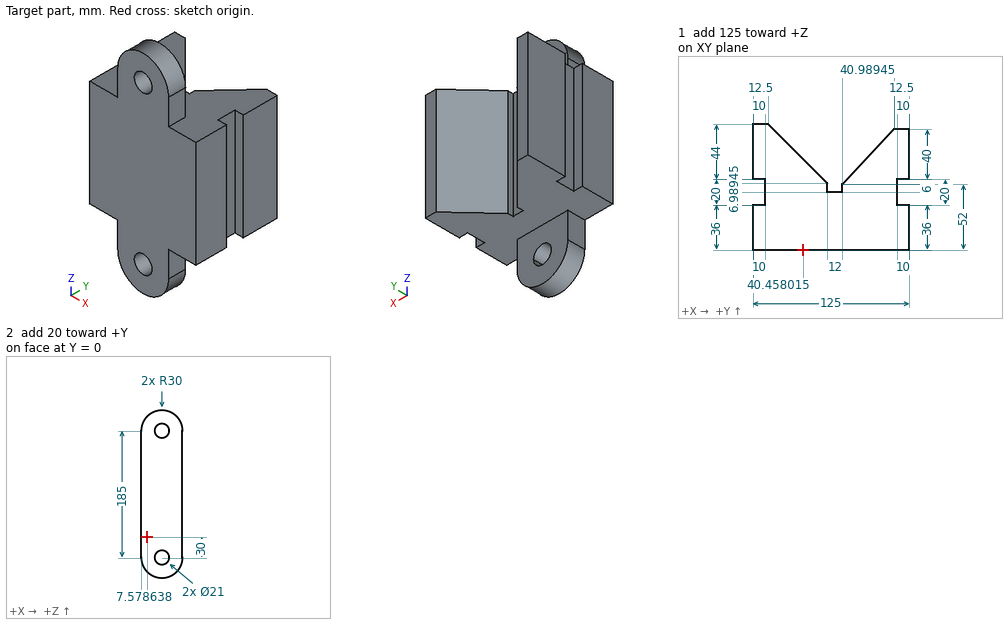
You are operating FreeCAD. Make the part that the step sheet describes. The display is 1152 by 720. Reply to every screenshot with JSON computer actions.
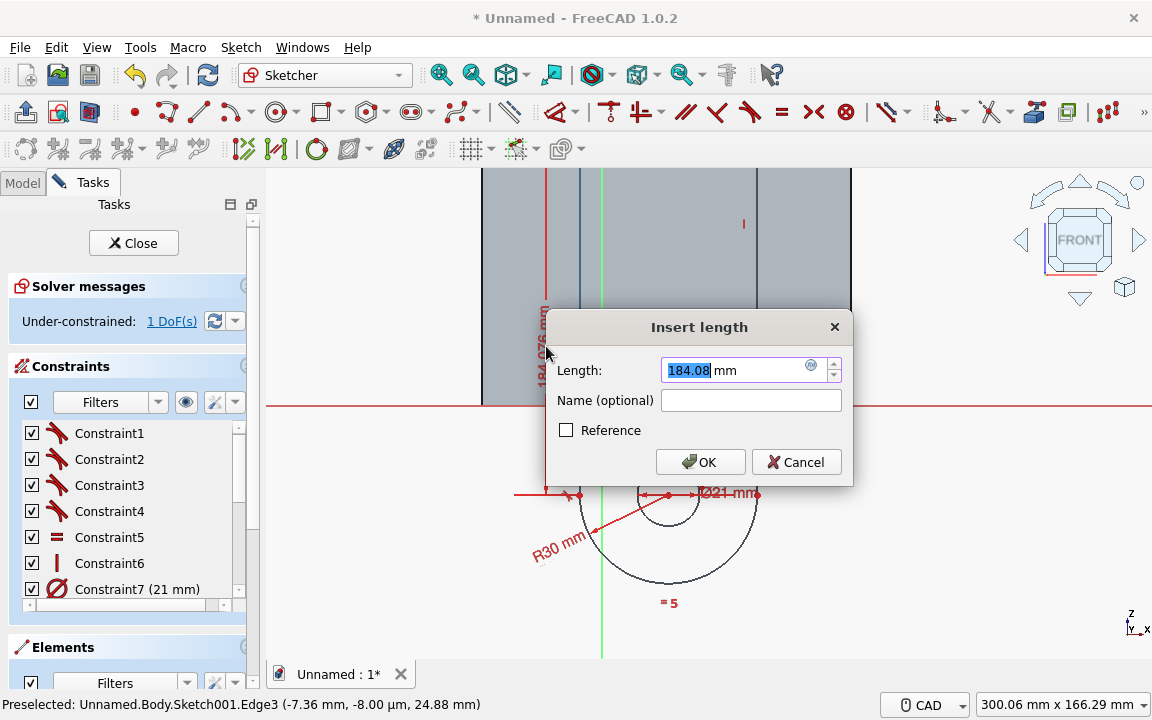
{"action": "type", "text": "185"}
{"action": "key", "text": "Return"}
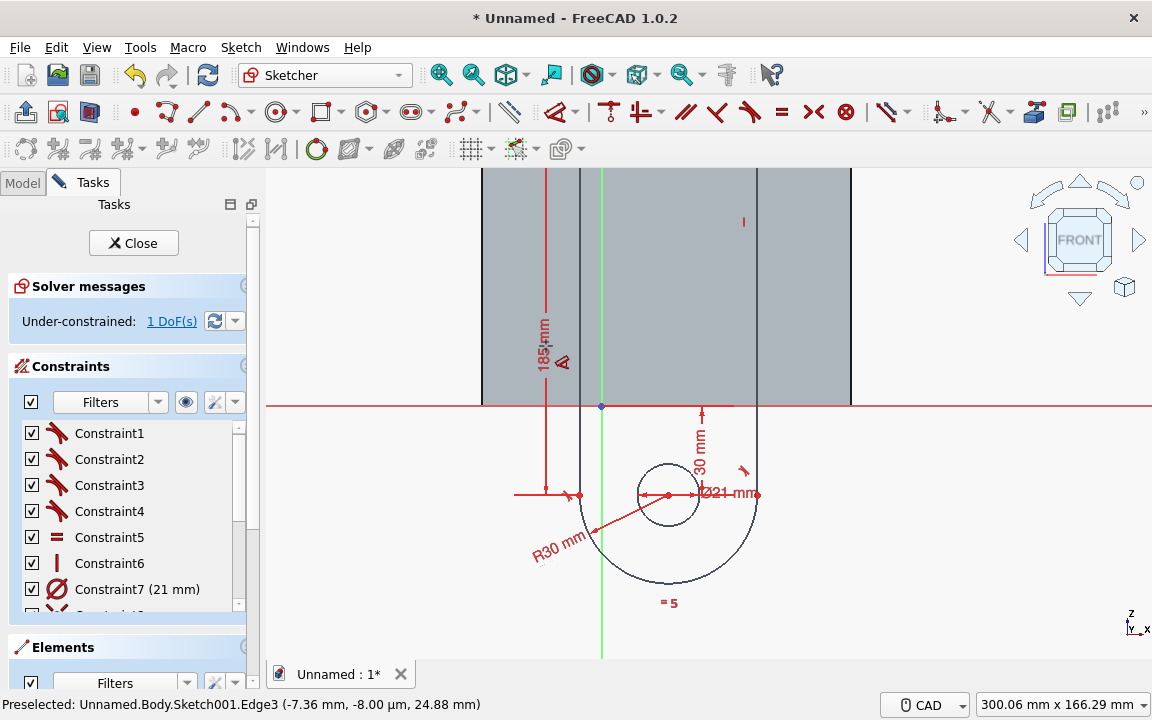
{"action": "scroll", "coordinate": [580, 495], "scroll_direction": "up", "scroll_amount": 3}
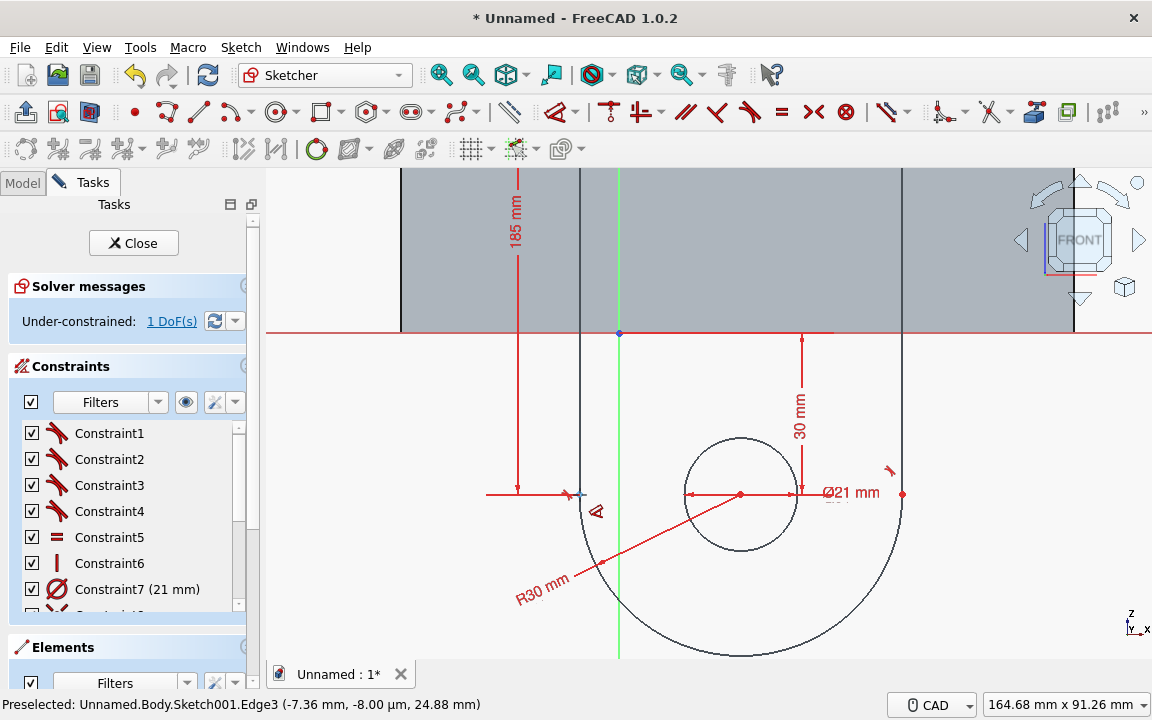
{"action": "left_click", "coordinate": [580, 495]}
{"action": "left_click", "coordinate": [599, 529]}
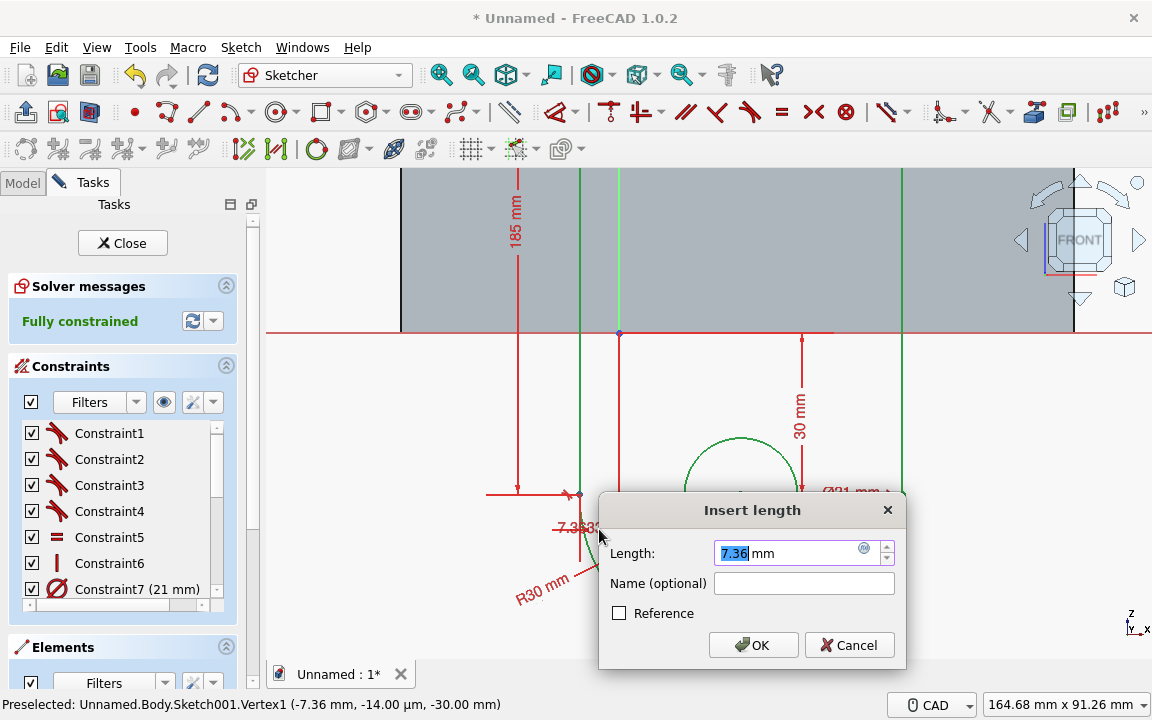
{"action": "type", "text": "7.578638"}
{"action": "key", "text": "Return"}
{"action": "key", "text": "Escape"}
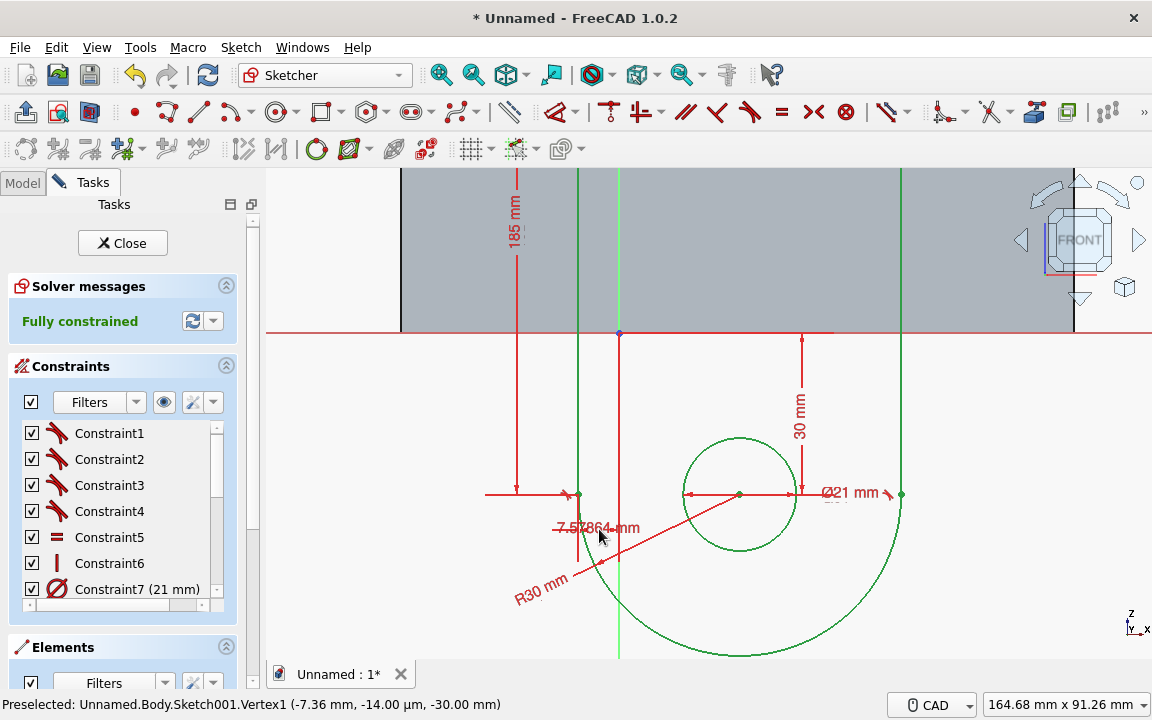
{"action": "left_click", "coordinate": [123, 243]}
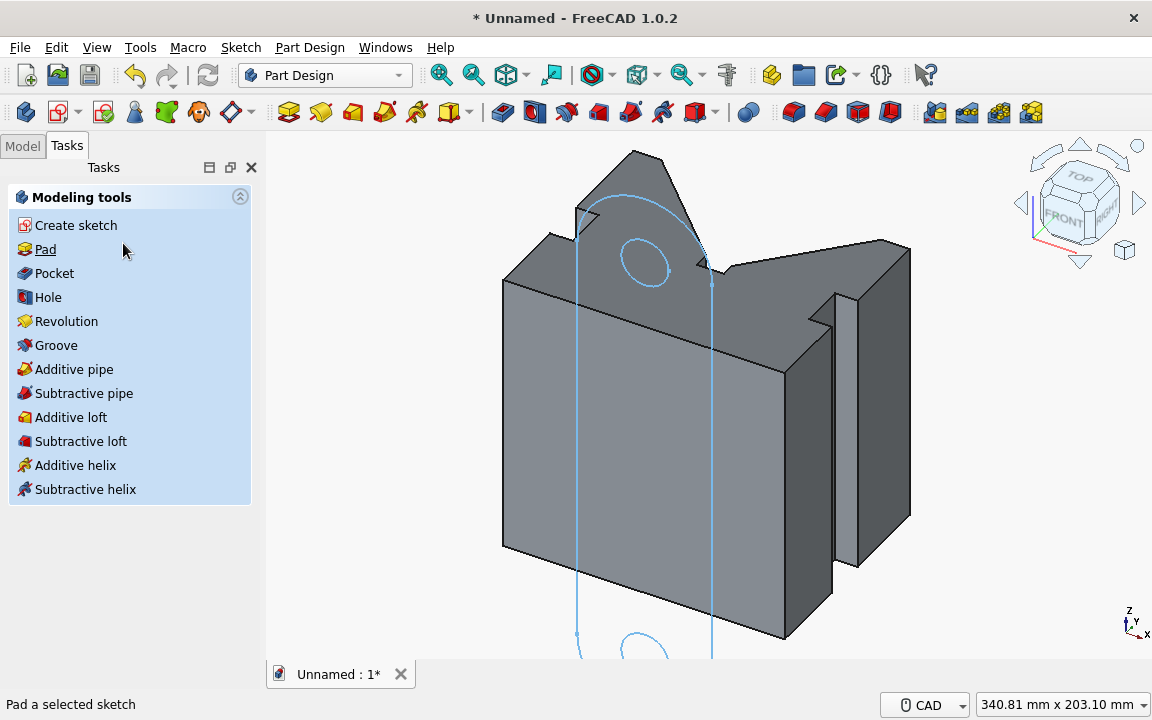
{"action": "left_click", "coordinate": [290, 112]}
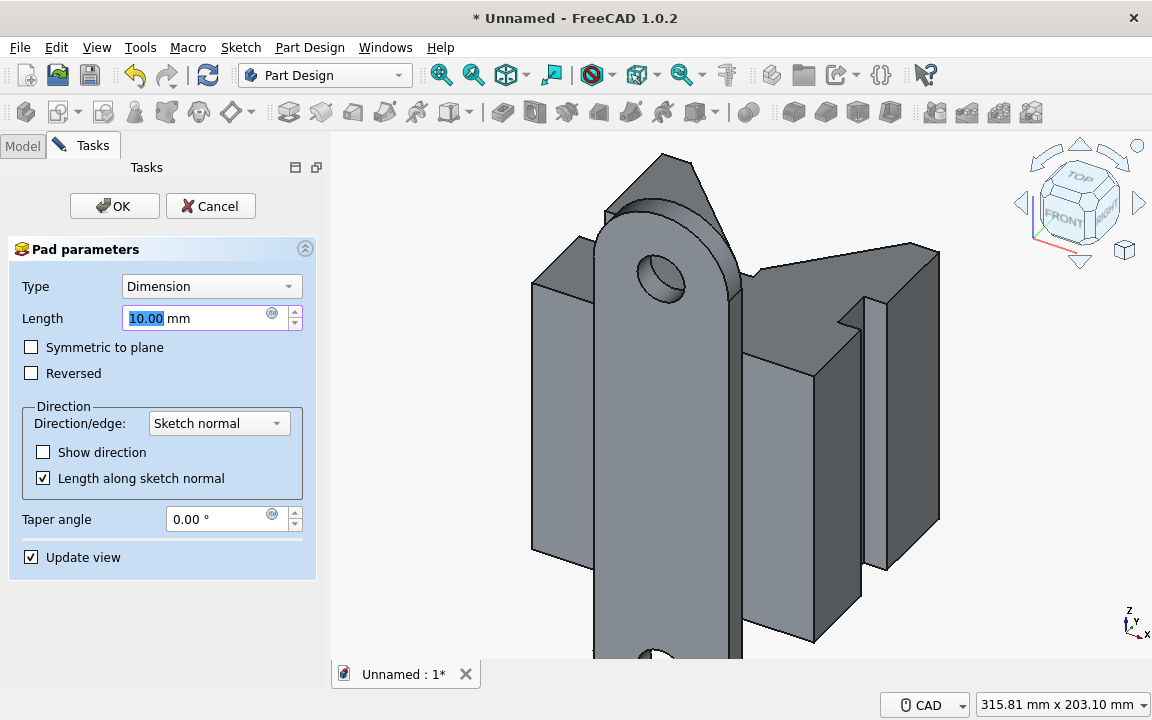
{"action": "type", "text": "20"}
{"action": "key", "text": "Tab"}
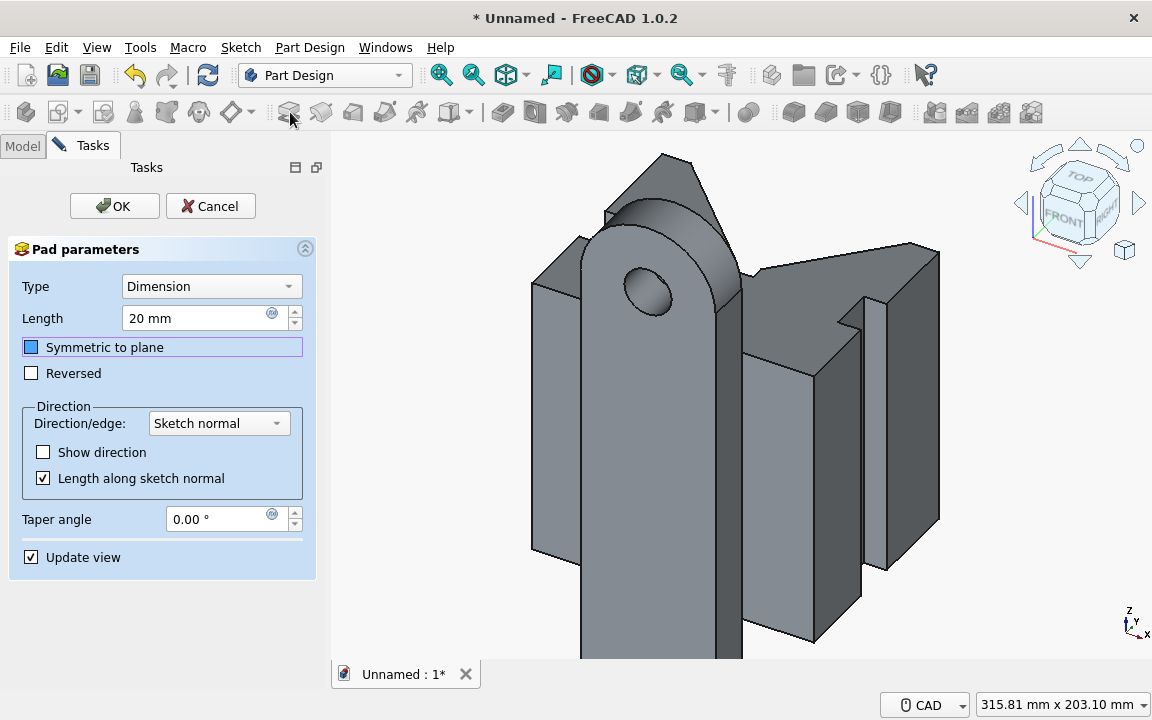
{"action": "left_click", "coordinate": [30, 373]}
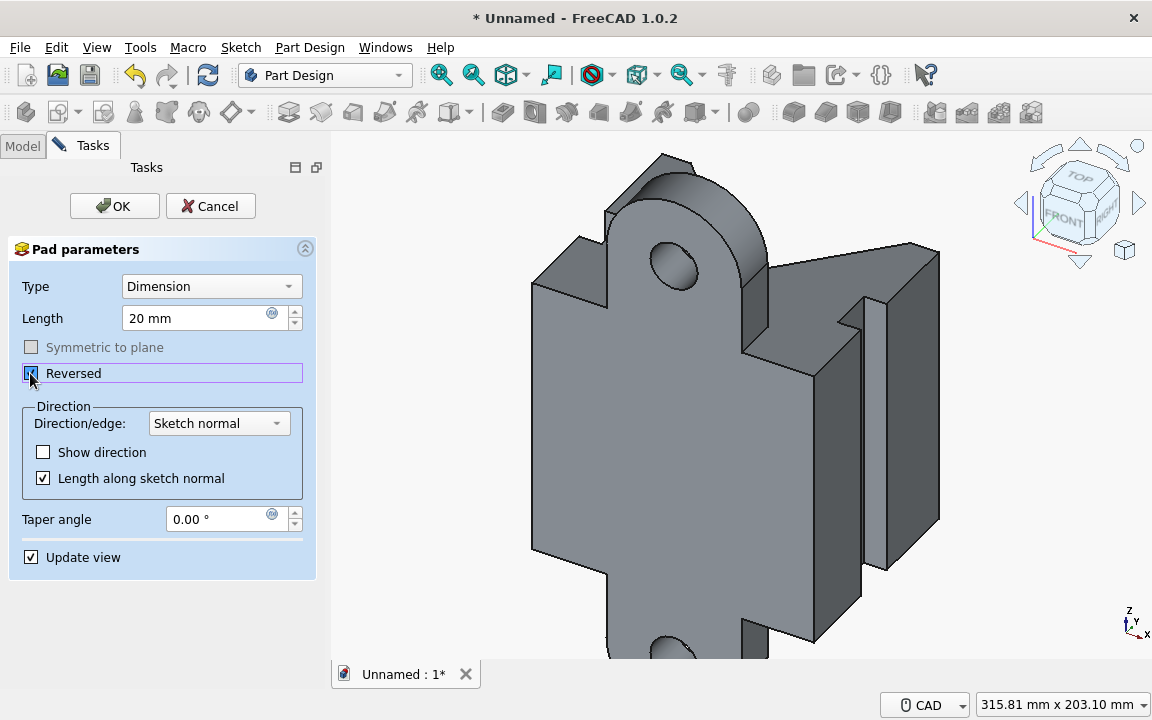
{"action": "left_click", "coordinate": [115, 206]}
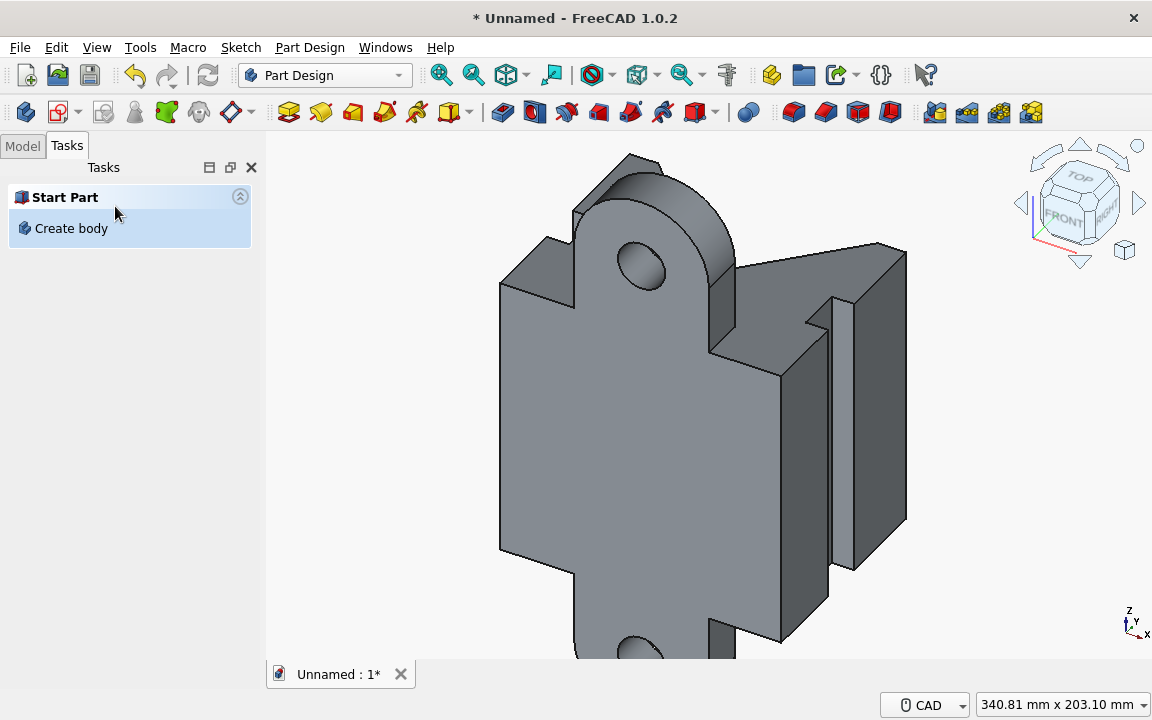
{"action": "key", "text": "0"}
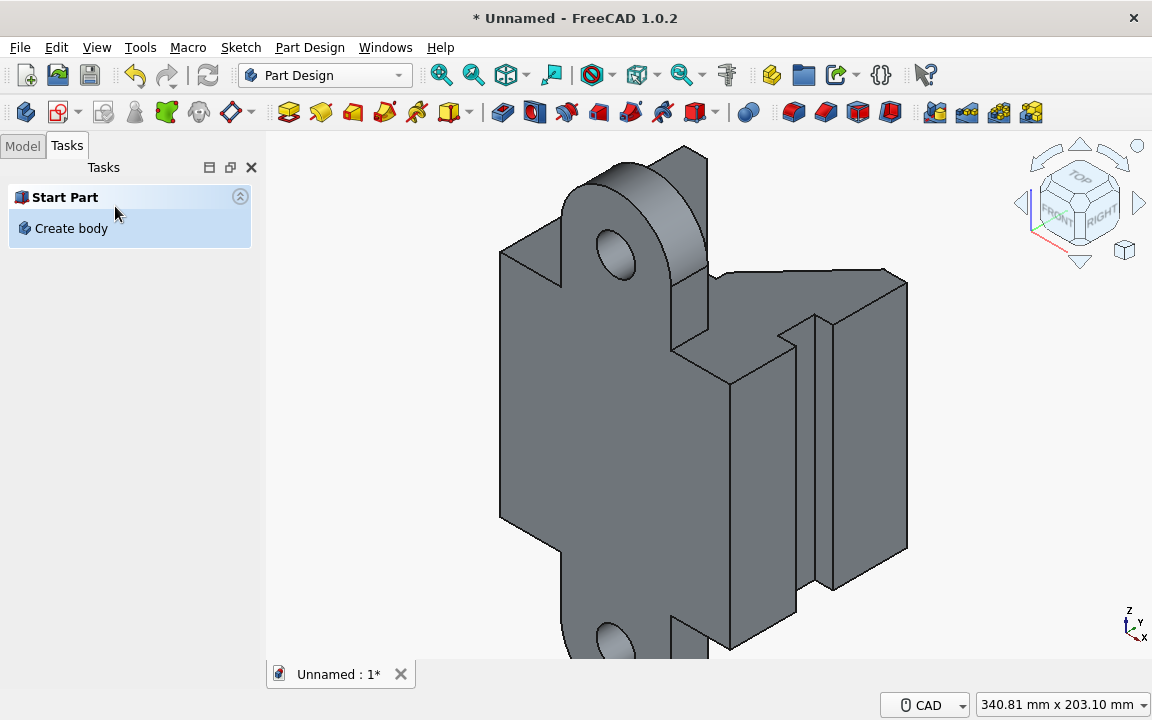
{"action": "key", "text": "v f"}